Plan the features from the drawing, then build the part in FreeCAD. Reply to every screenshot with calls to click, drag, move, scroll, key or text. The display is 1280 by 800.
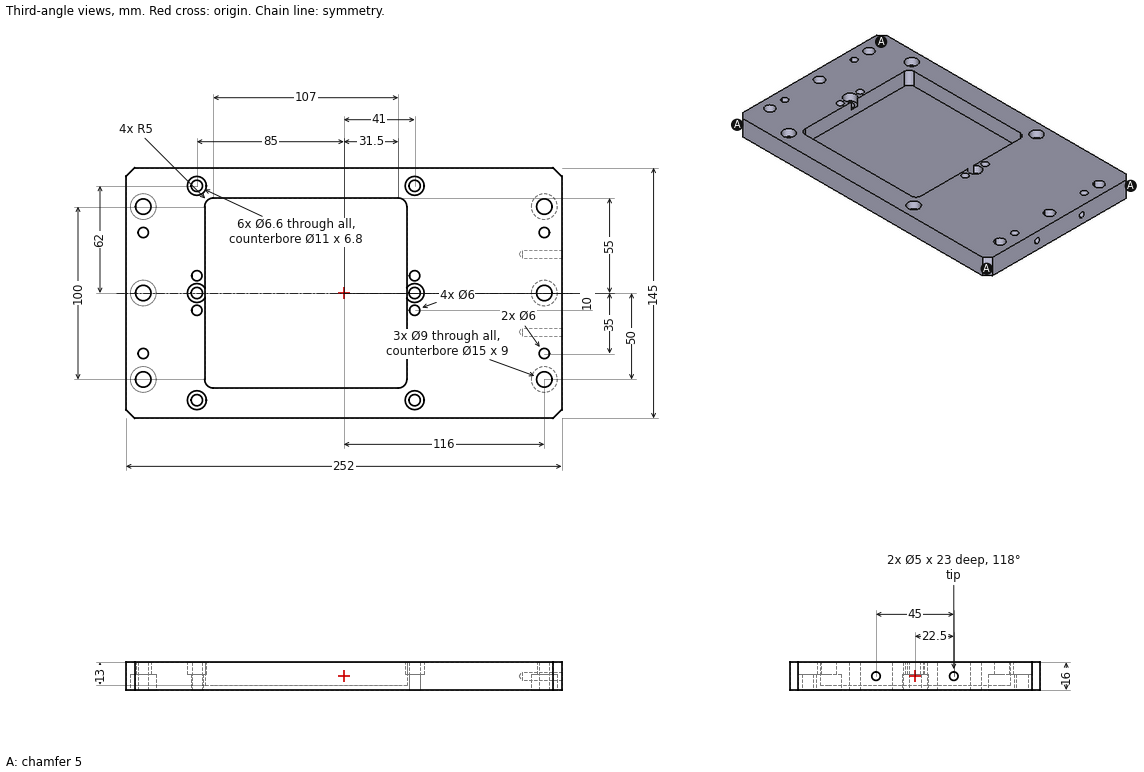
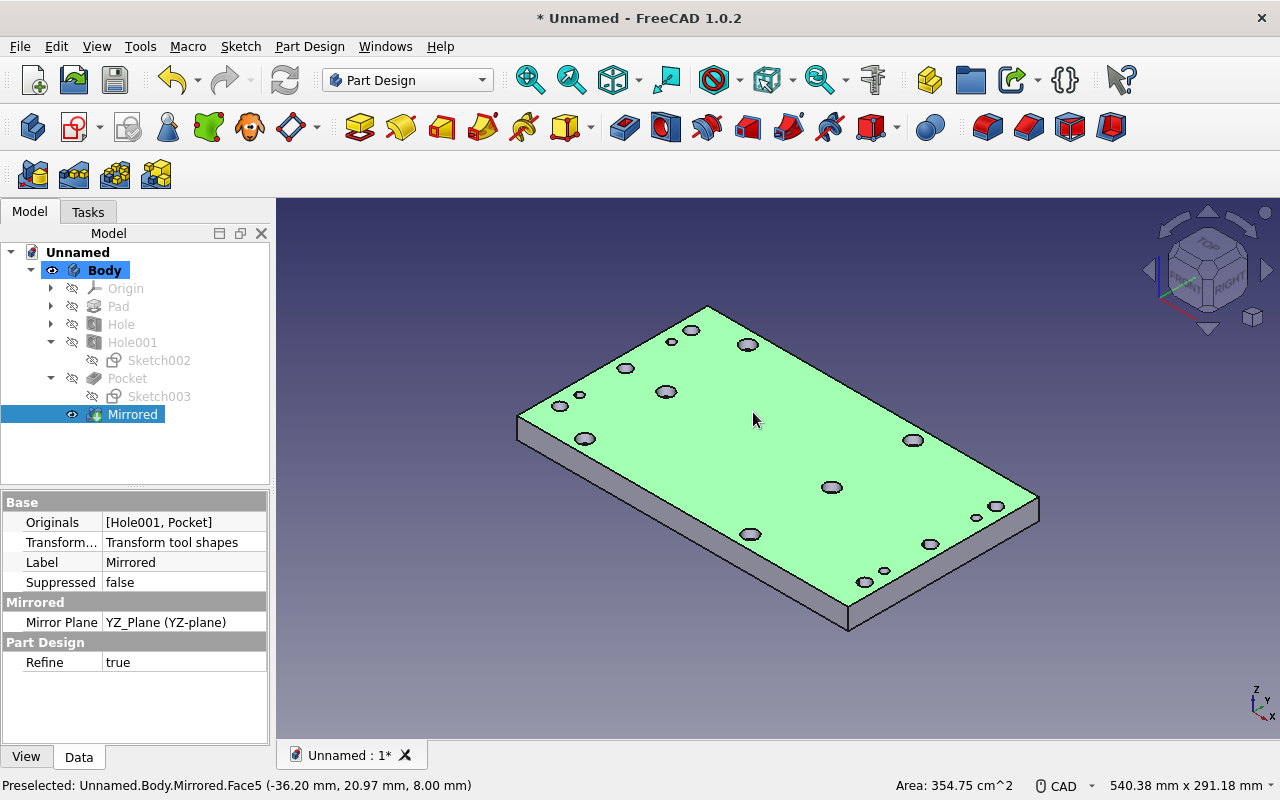
click(74, 128)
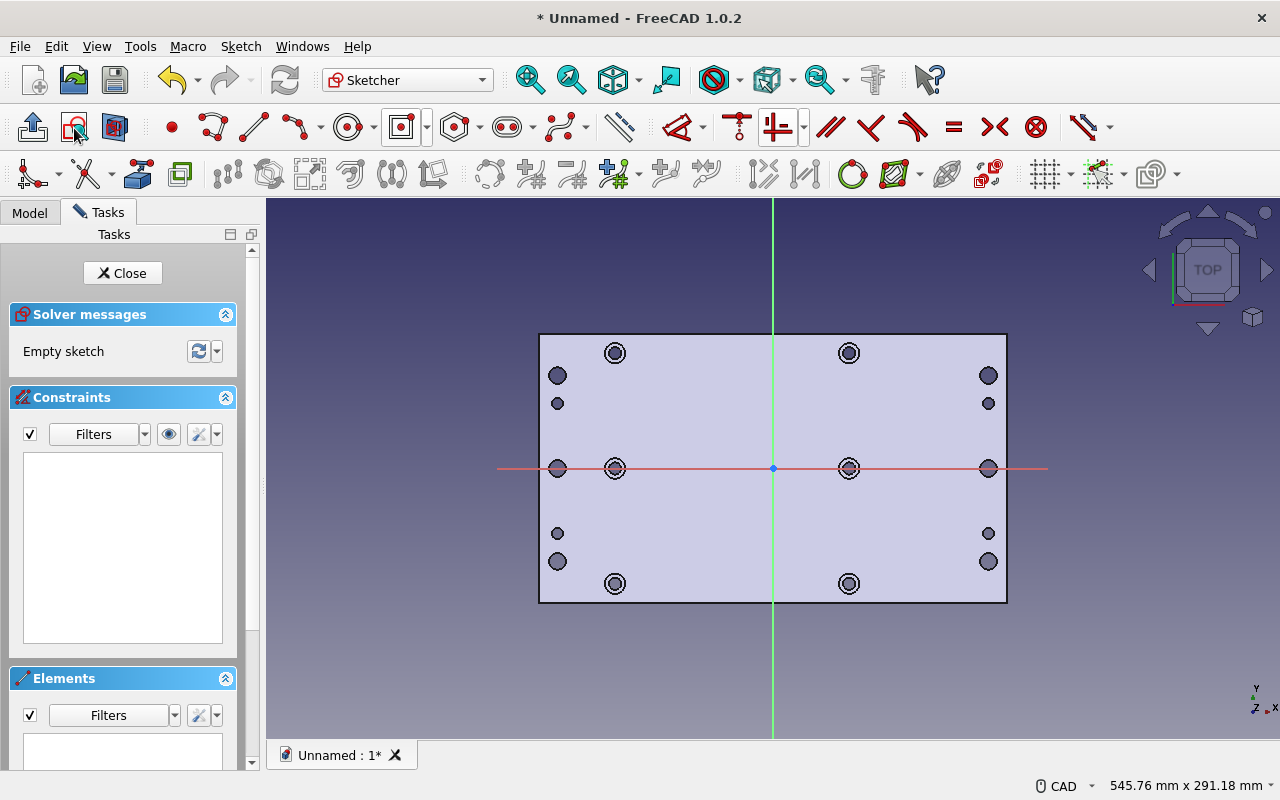
scroll(755, 468, up, 4)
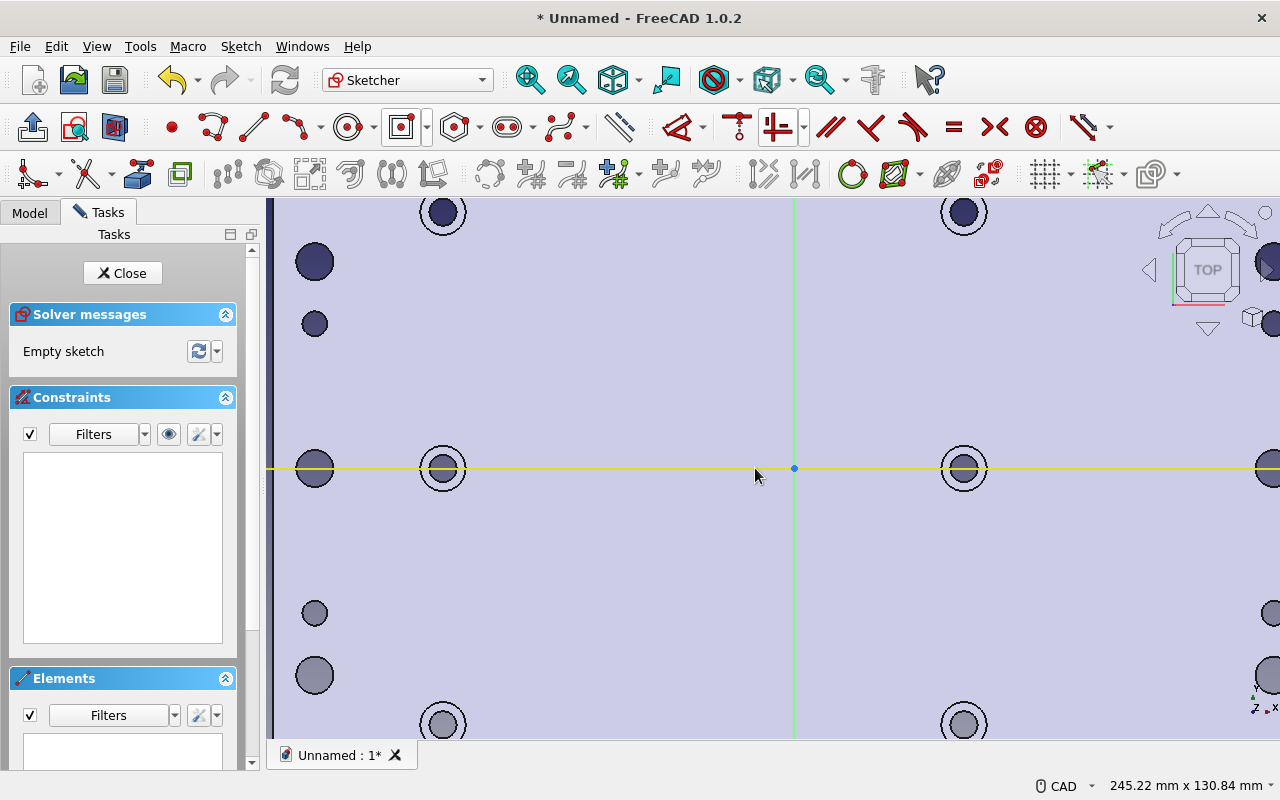
key(g)
key(c)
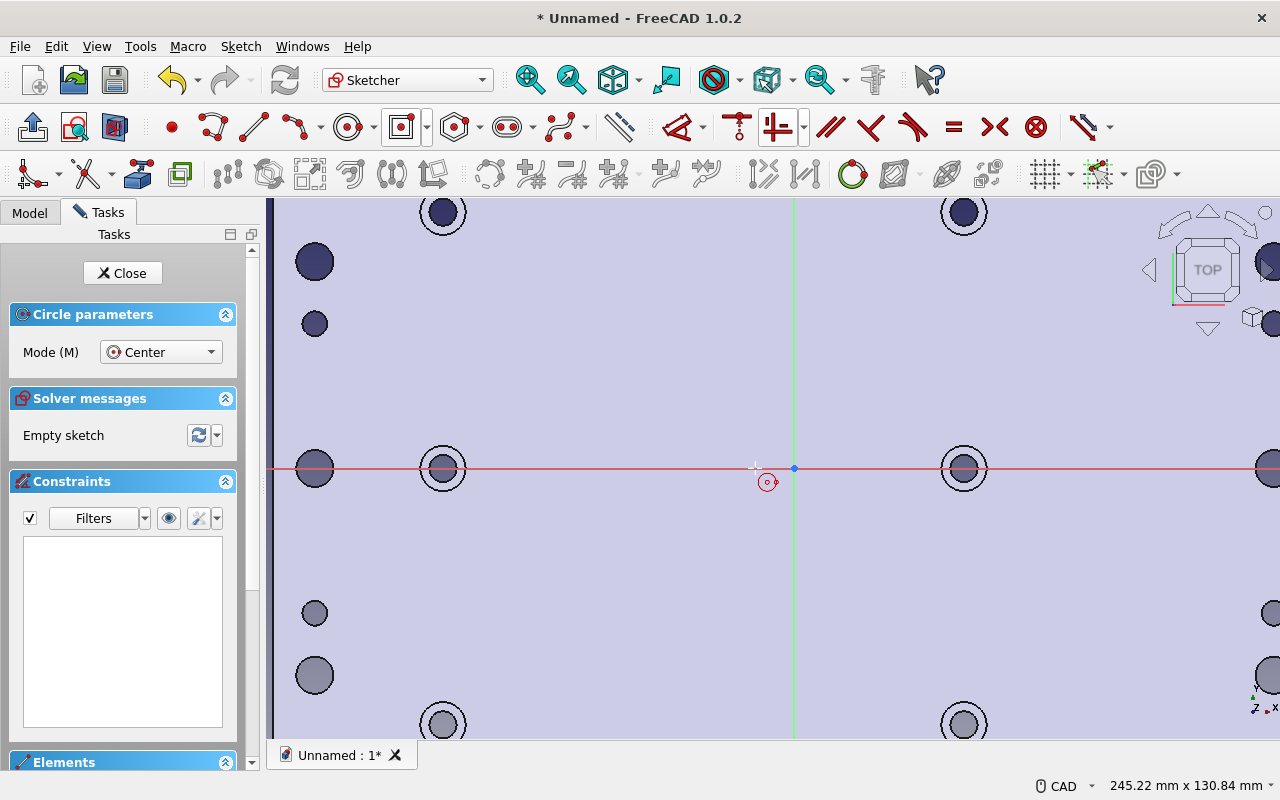
scroll(964, 510, up, 4)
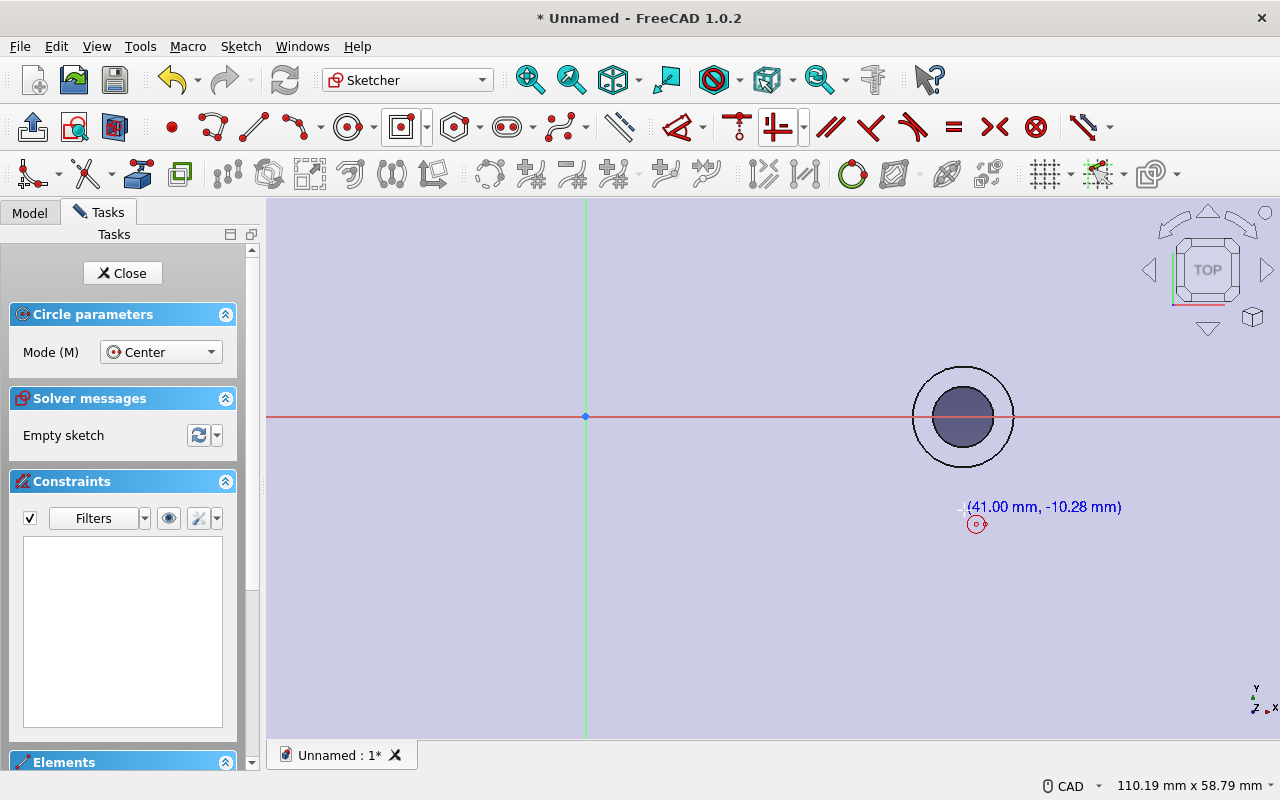
click(963, 509)
move(983, 489)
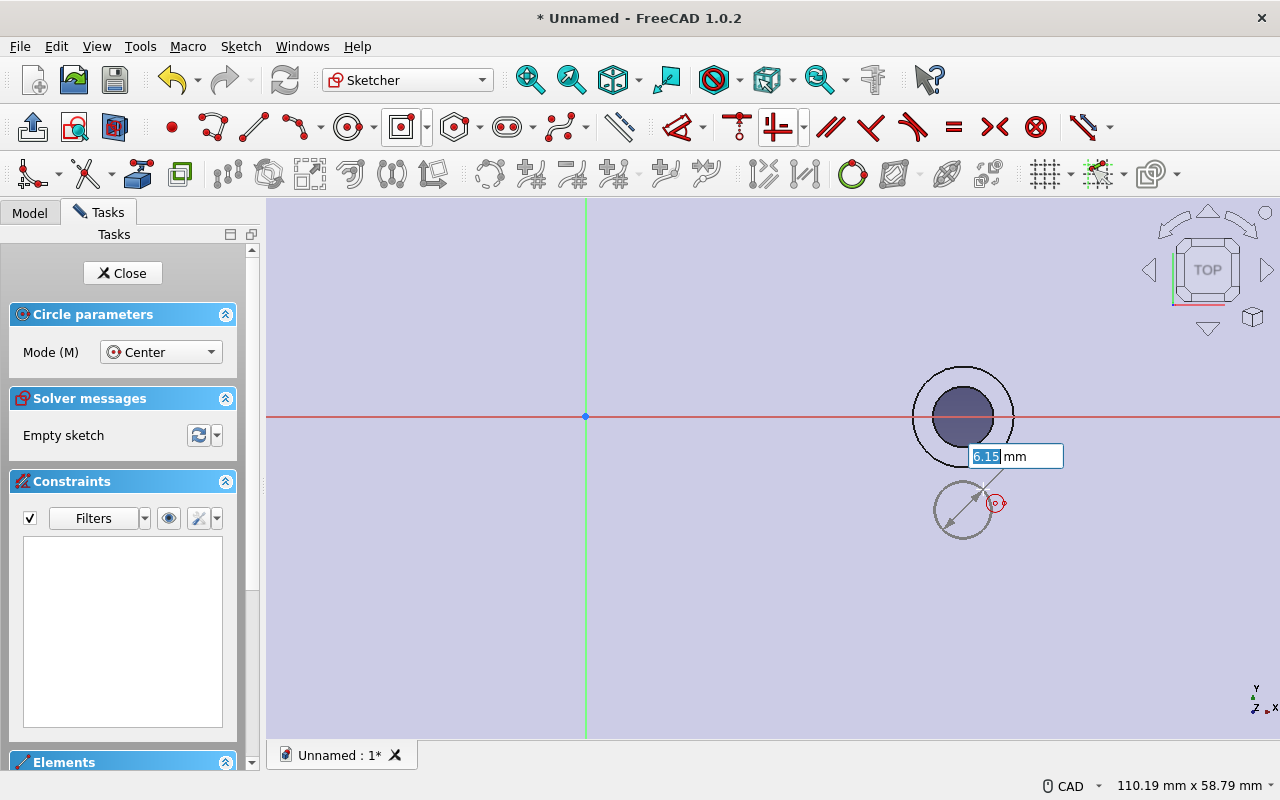
text(6)
key(Return)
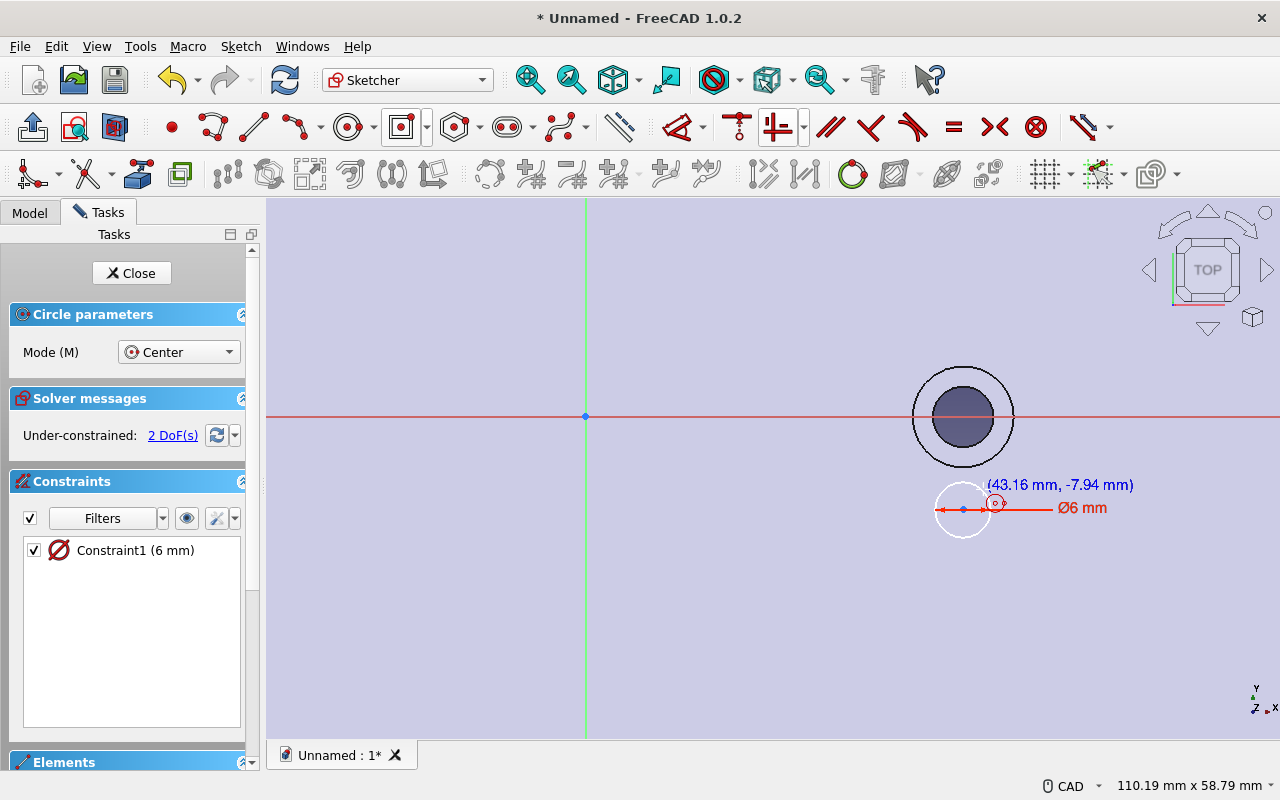
scroll(967, 511, down, 4)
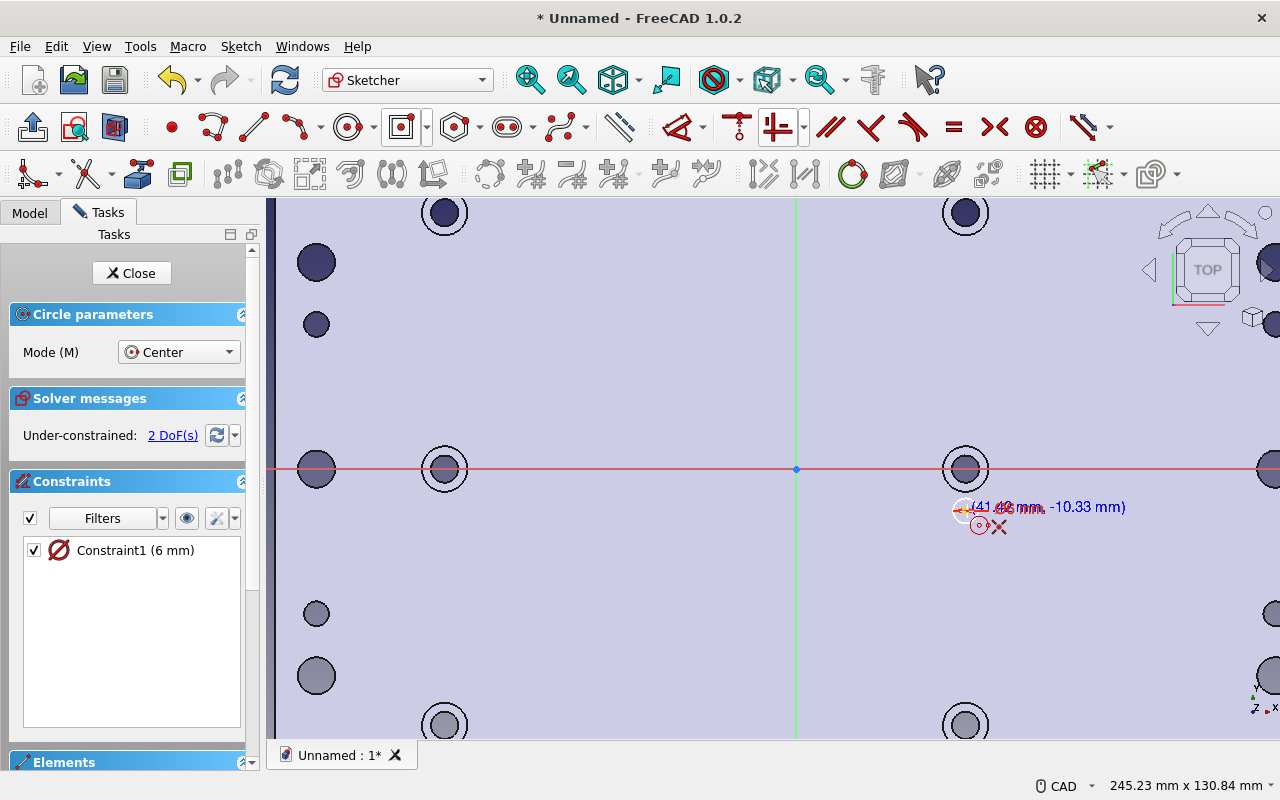
scroll(445, 510, up, 4)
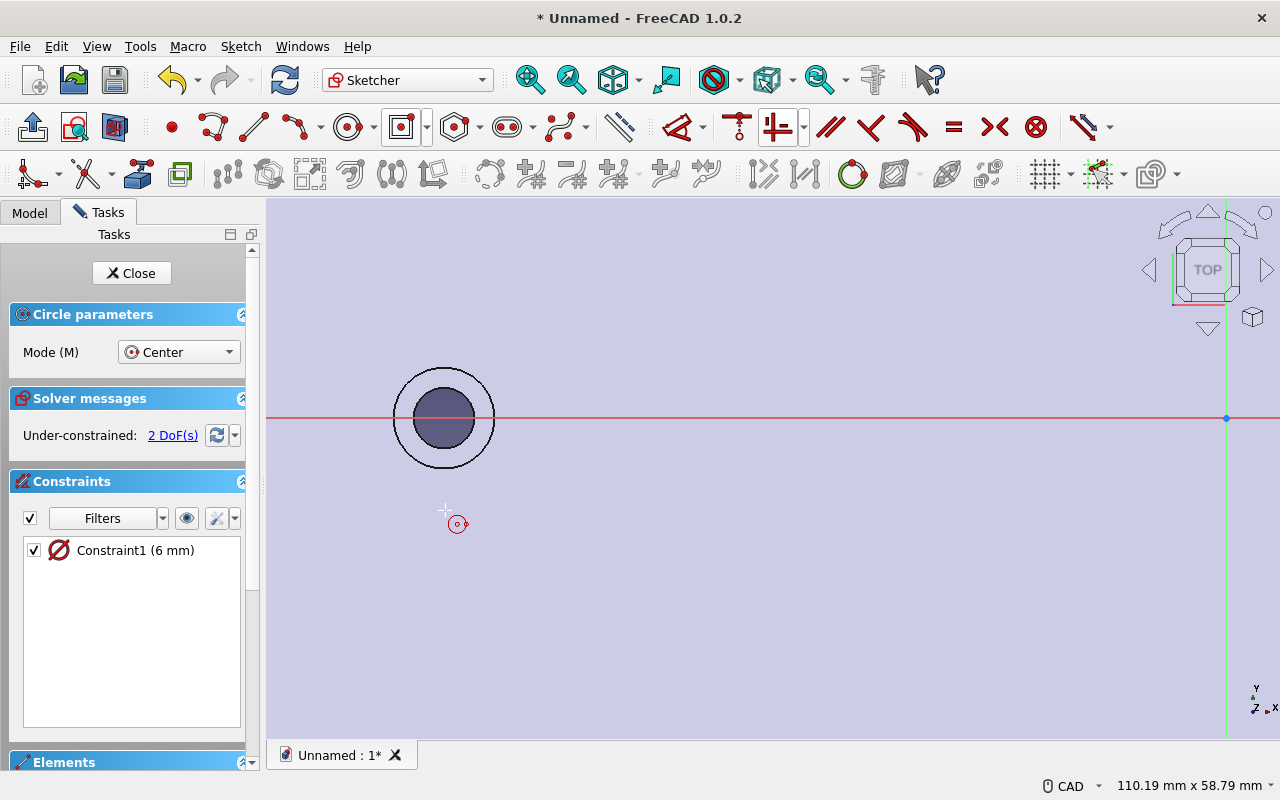
click(444, 510)
move(464, 491)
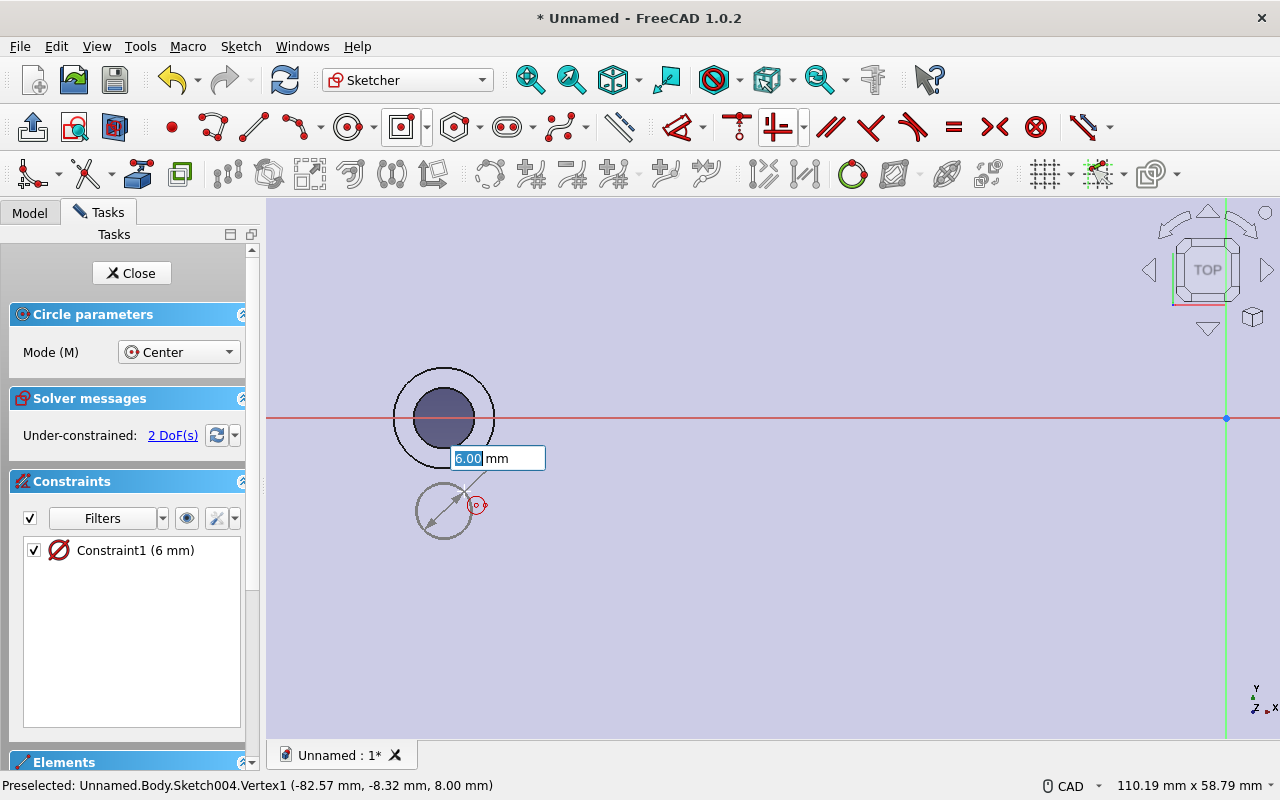
text(6)
key(Return)